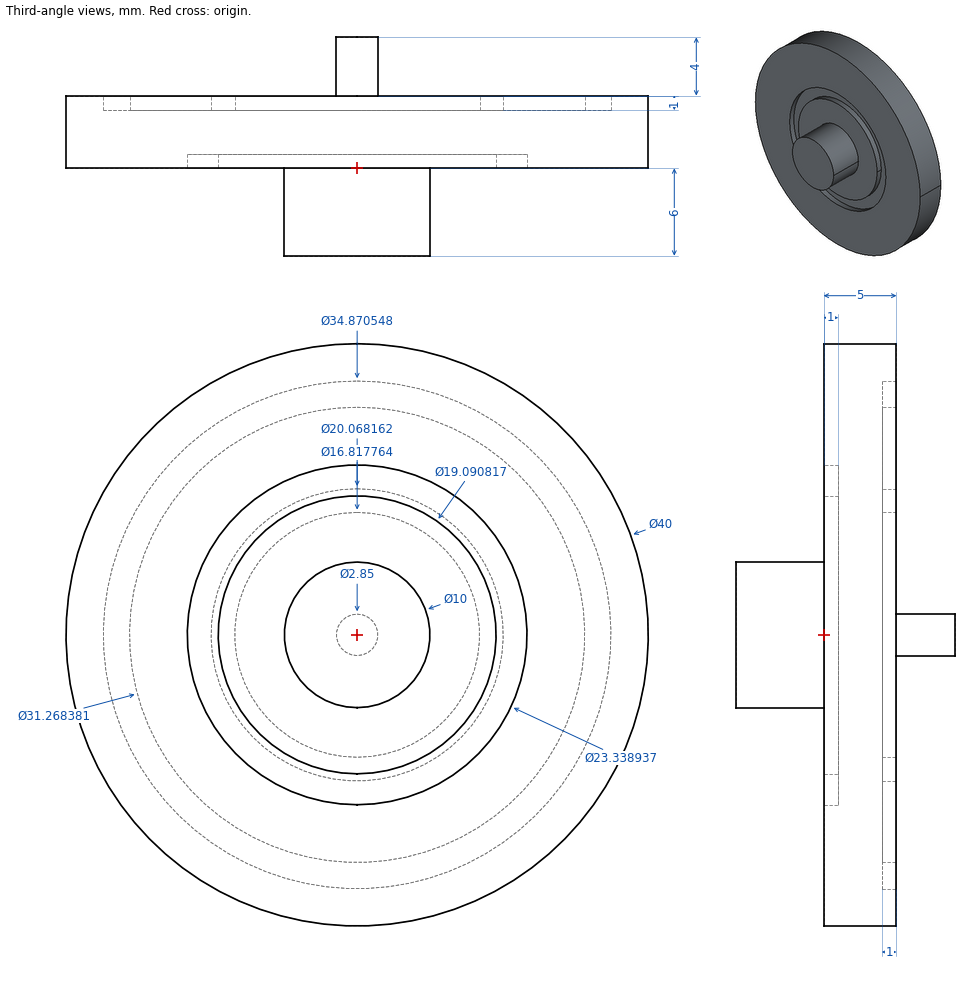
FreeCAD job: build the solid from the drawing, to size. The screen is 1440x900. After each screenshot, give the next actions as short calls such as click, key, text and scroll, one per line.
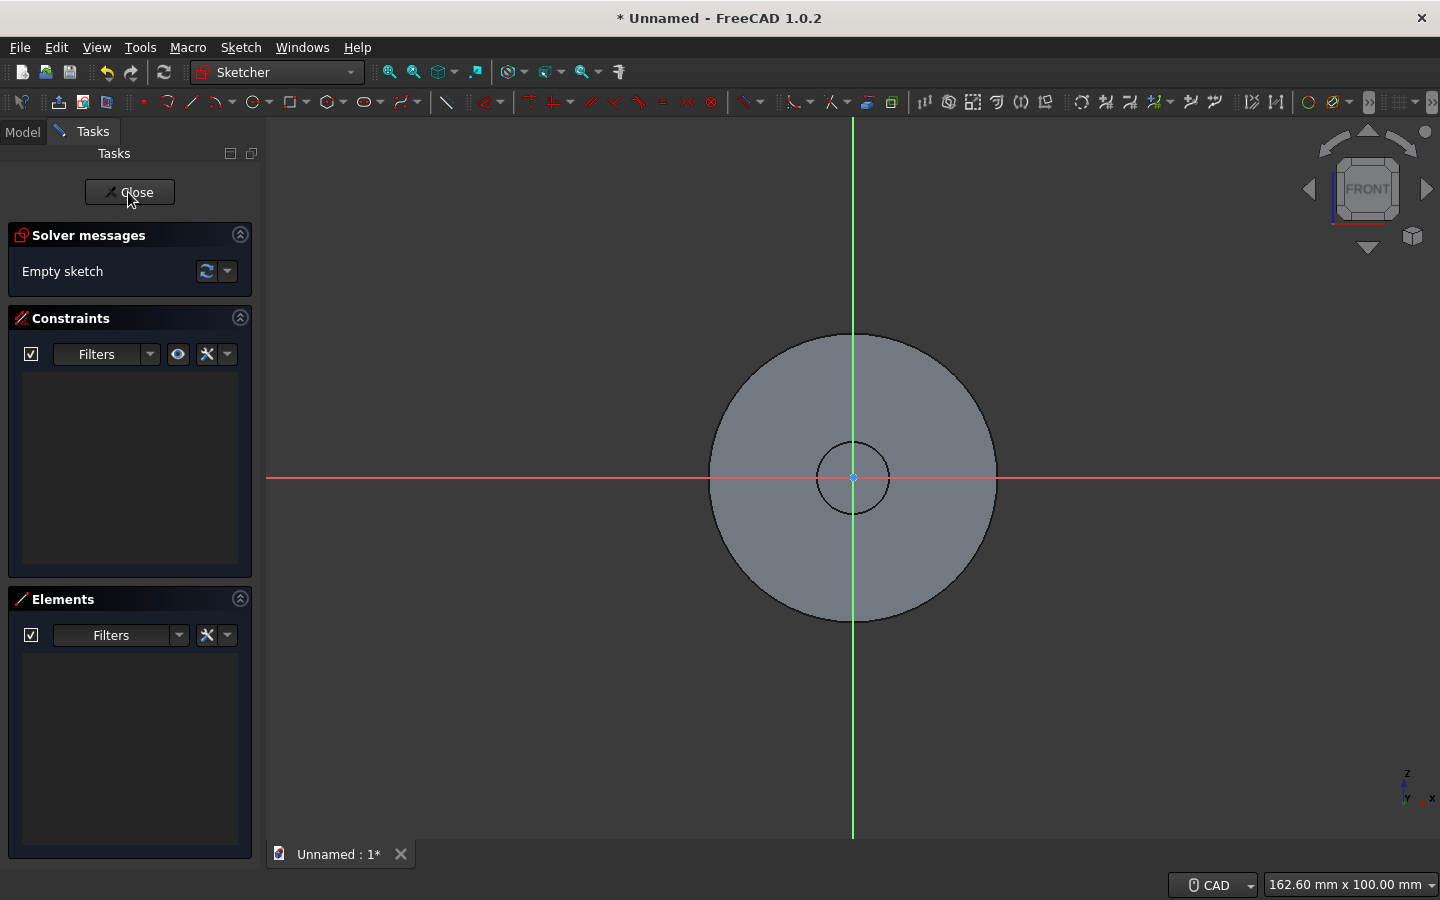
scroll(893, 478, up, 5)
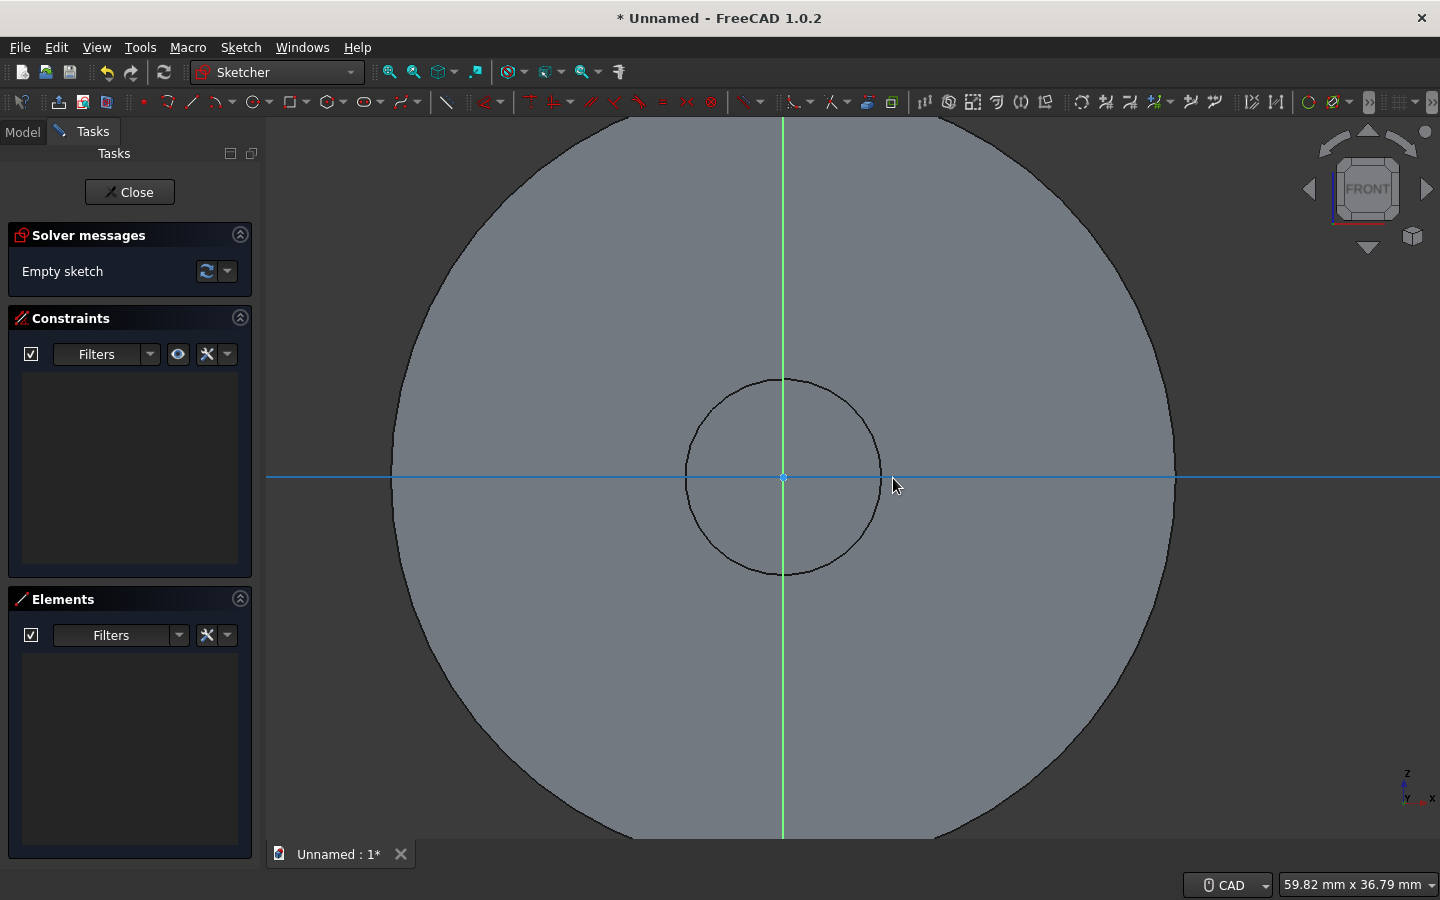
key(g)
key(c)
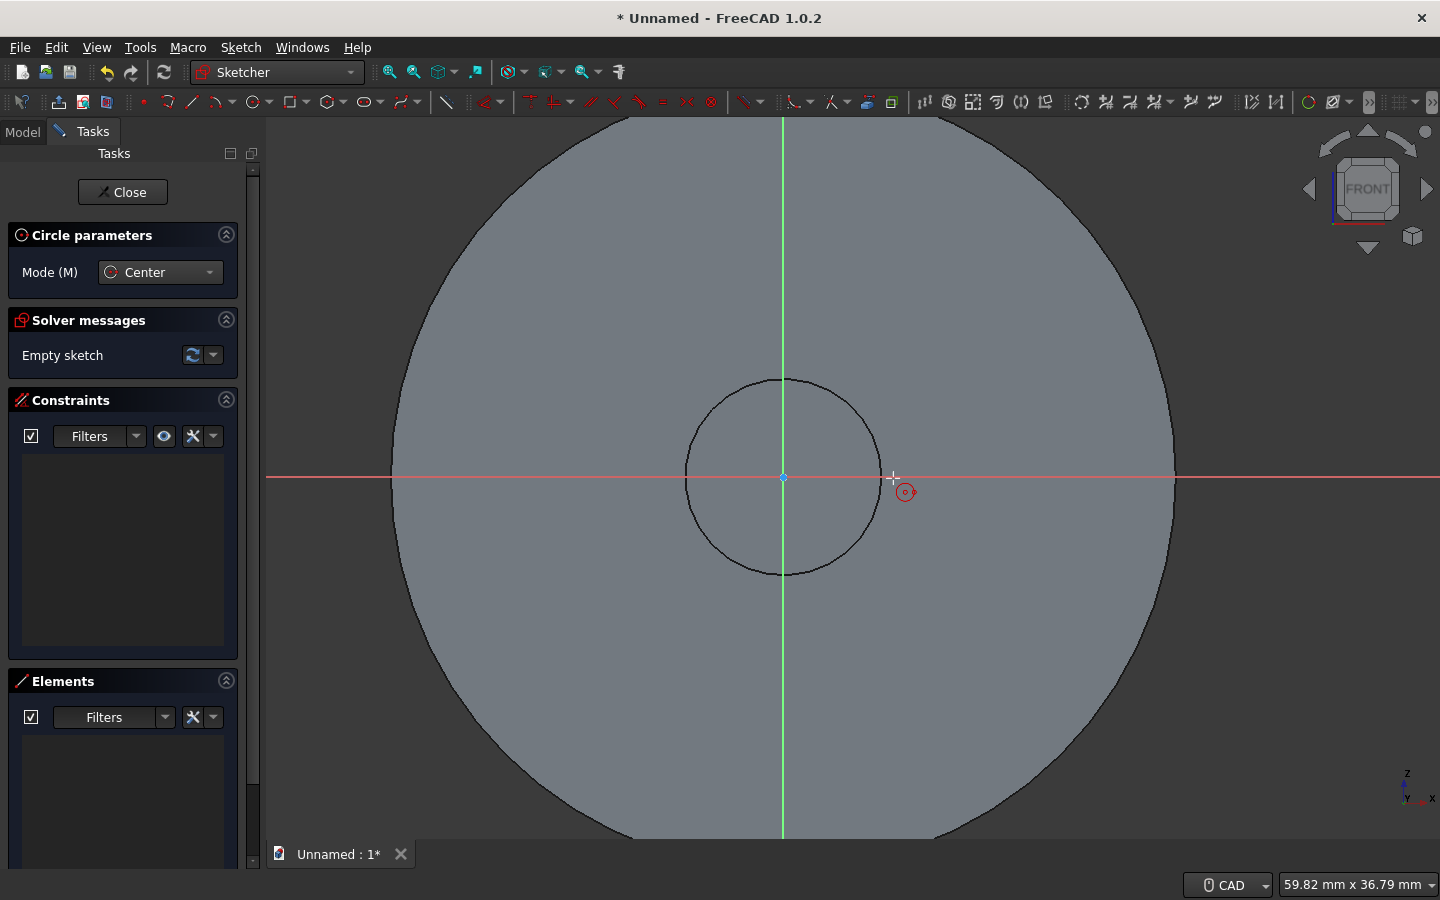
click(783, 477)
click(945, 315)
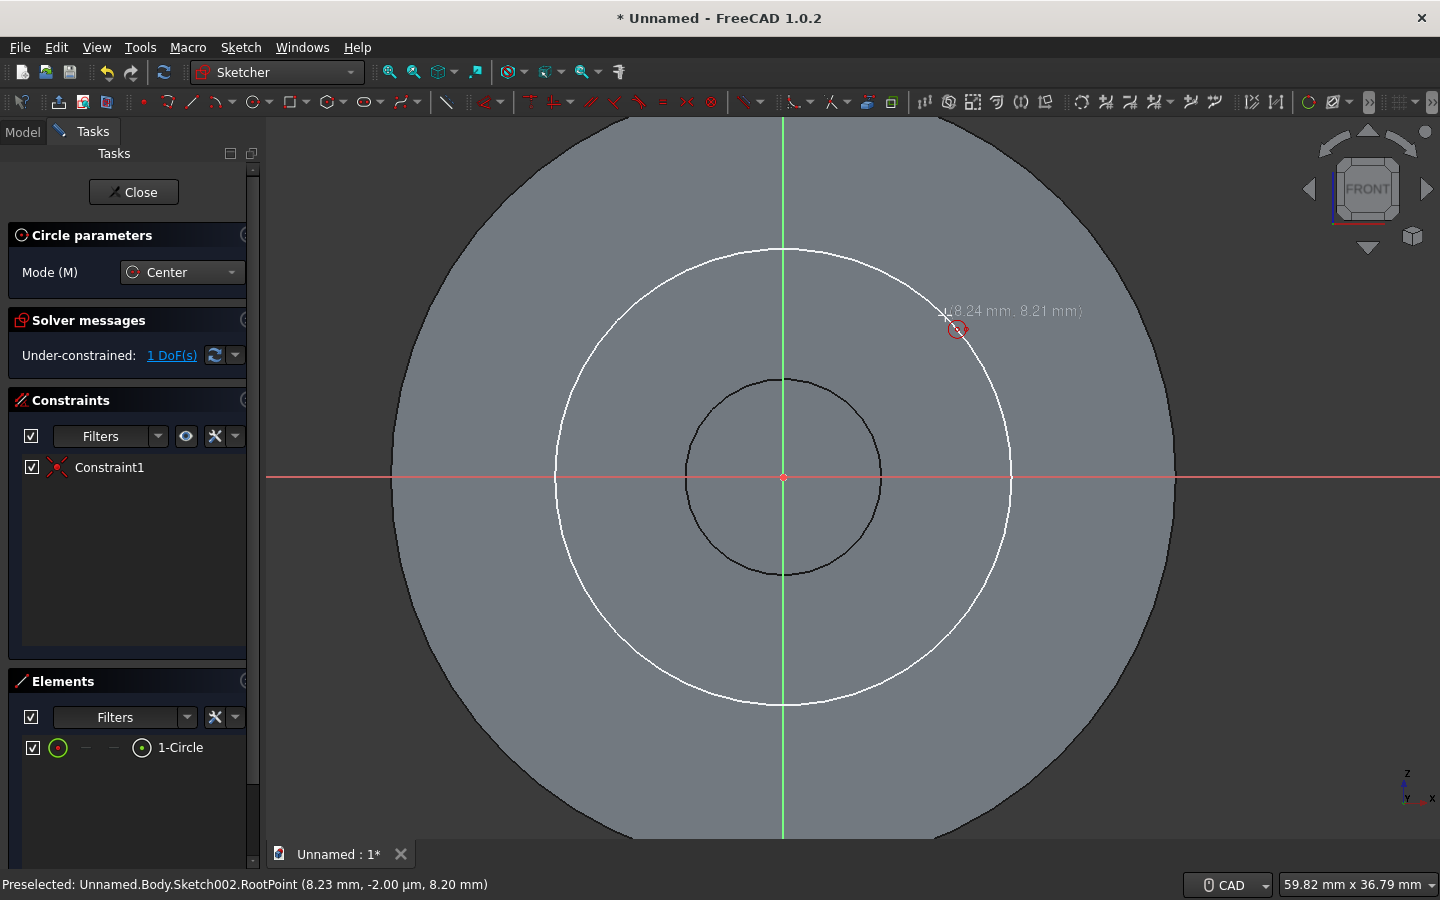
click(783, 477)
click(916, 345)
key(Escape)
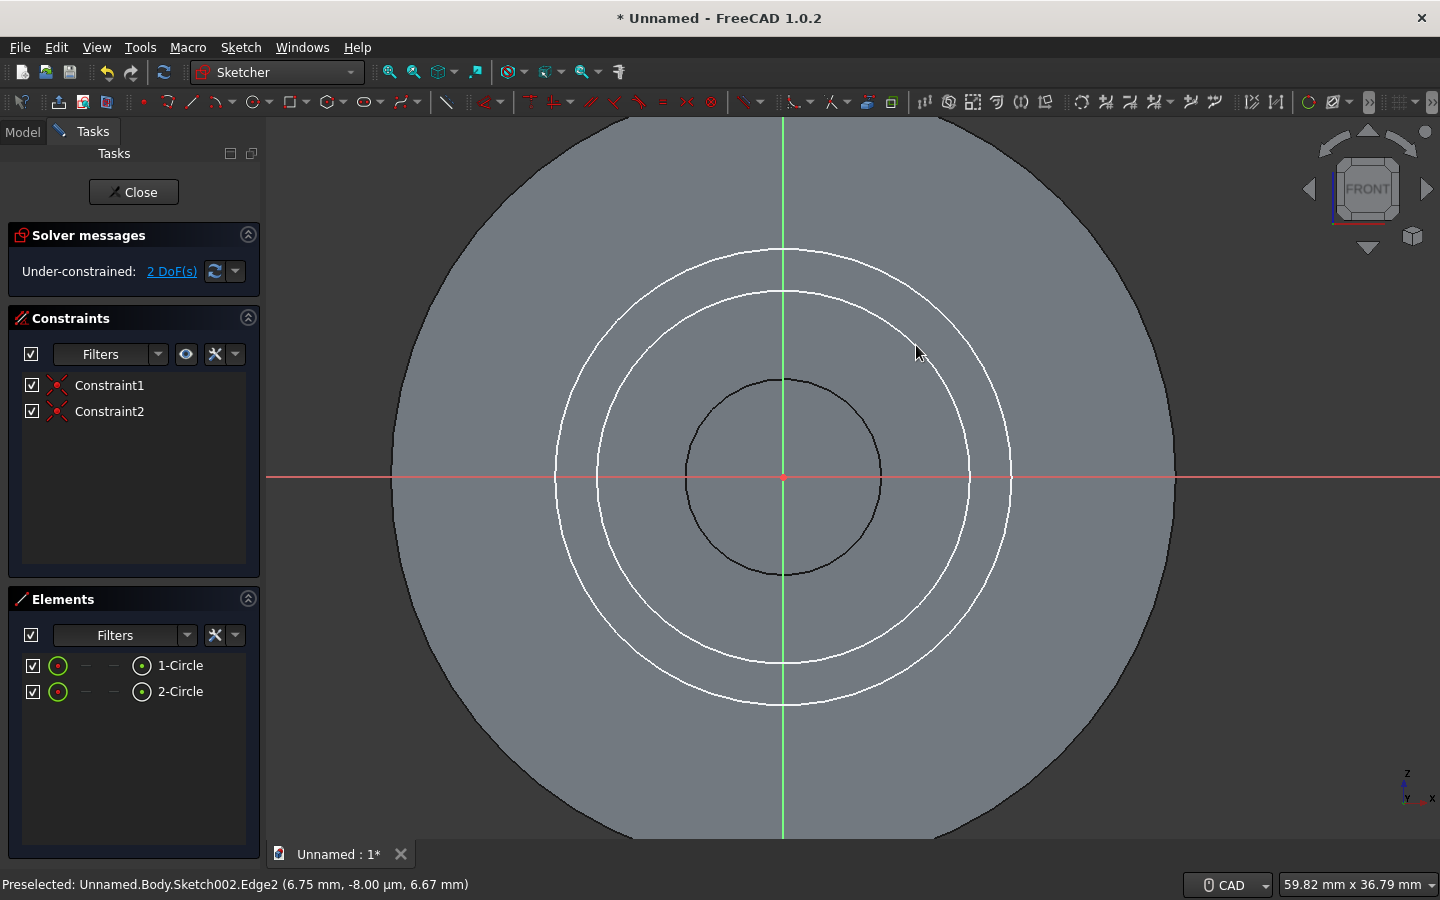
click(484, 102)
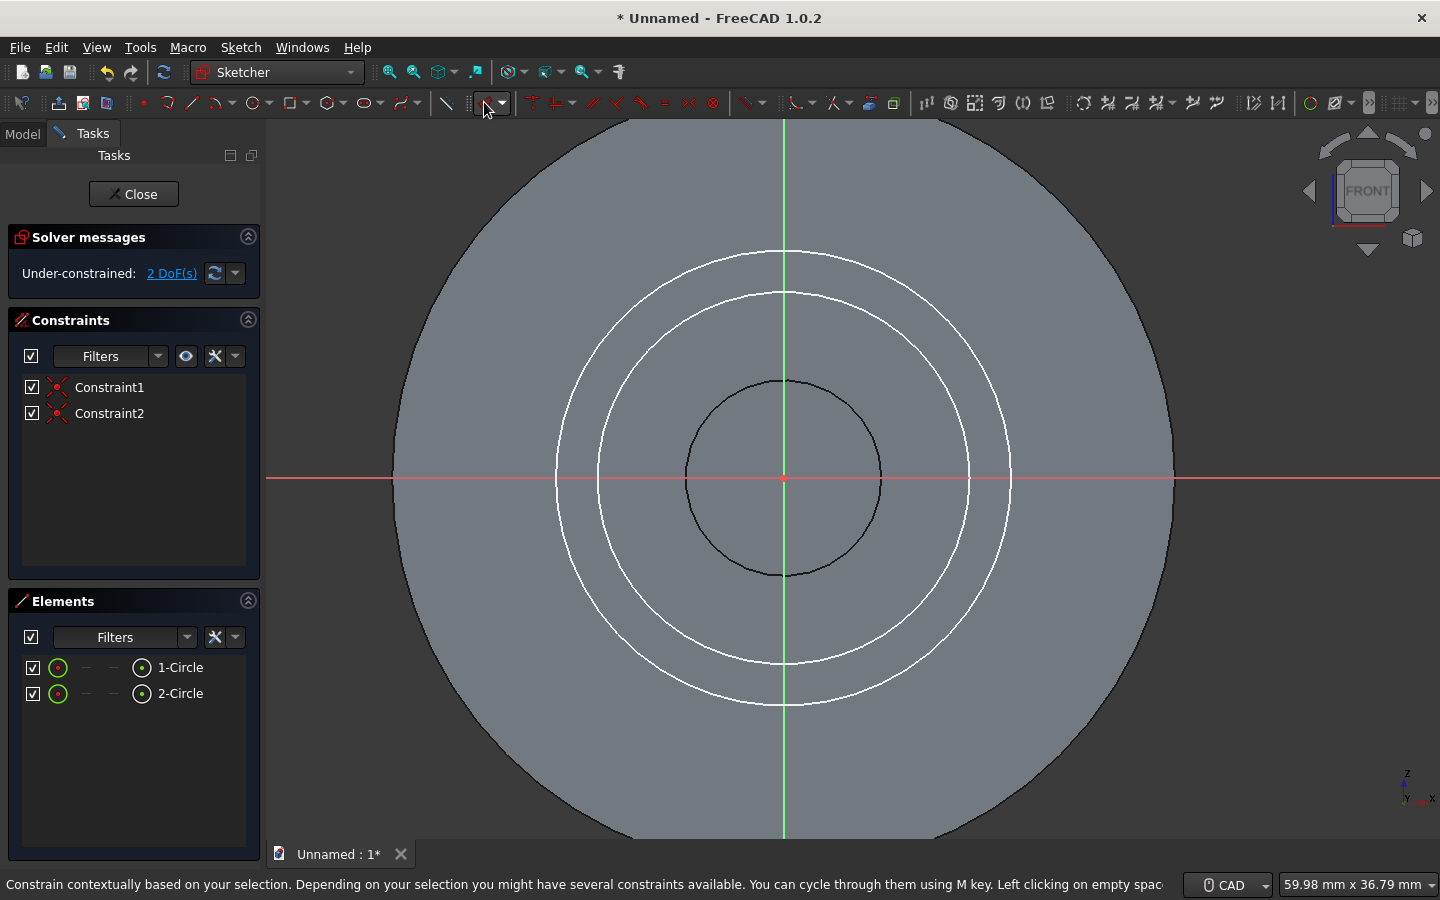
click(944, 317)
click(967, 294)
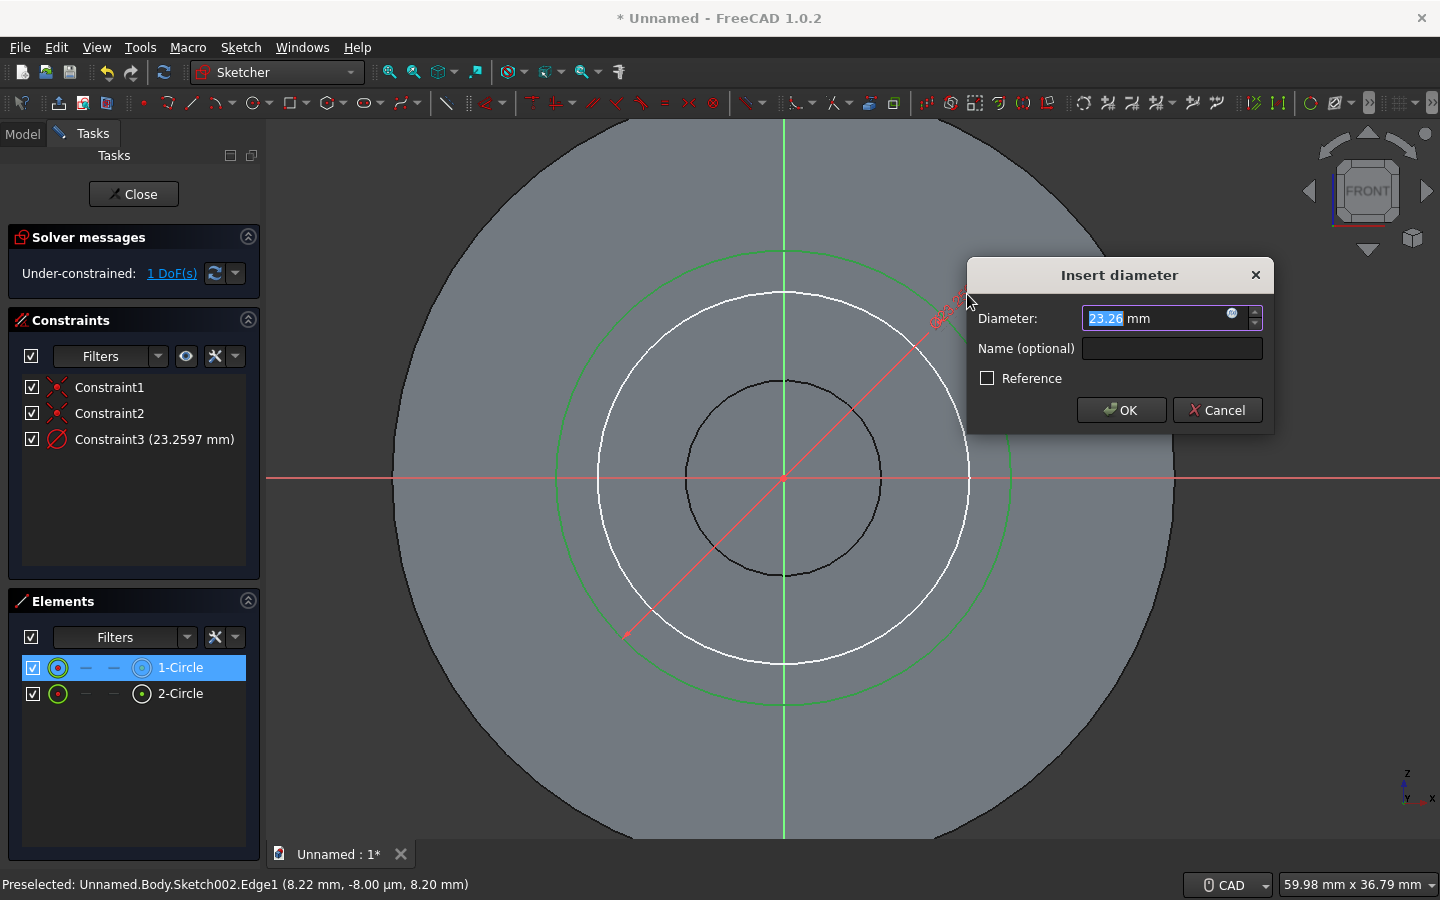
text(23.338937)
key(Return)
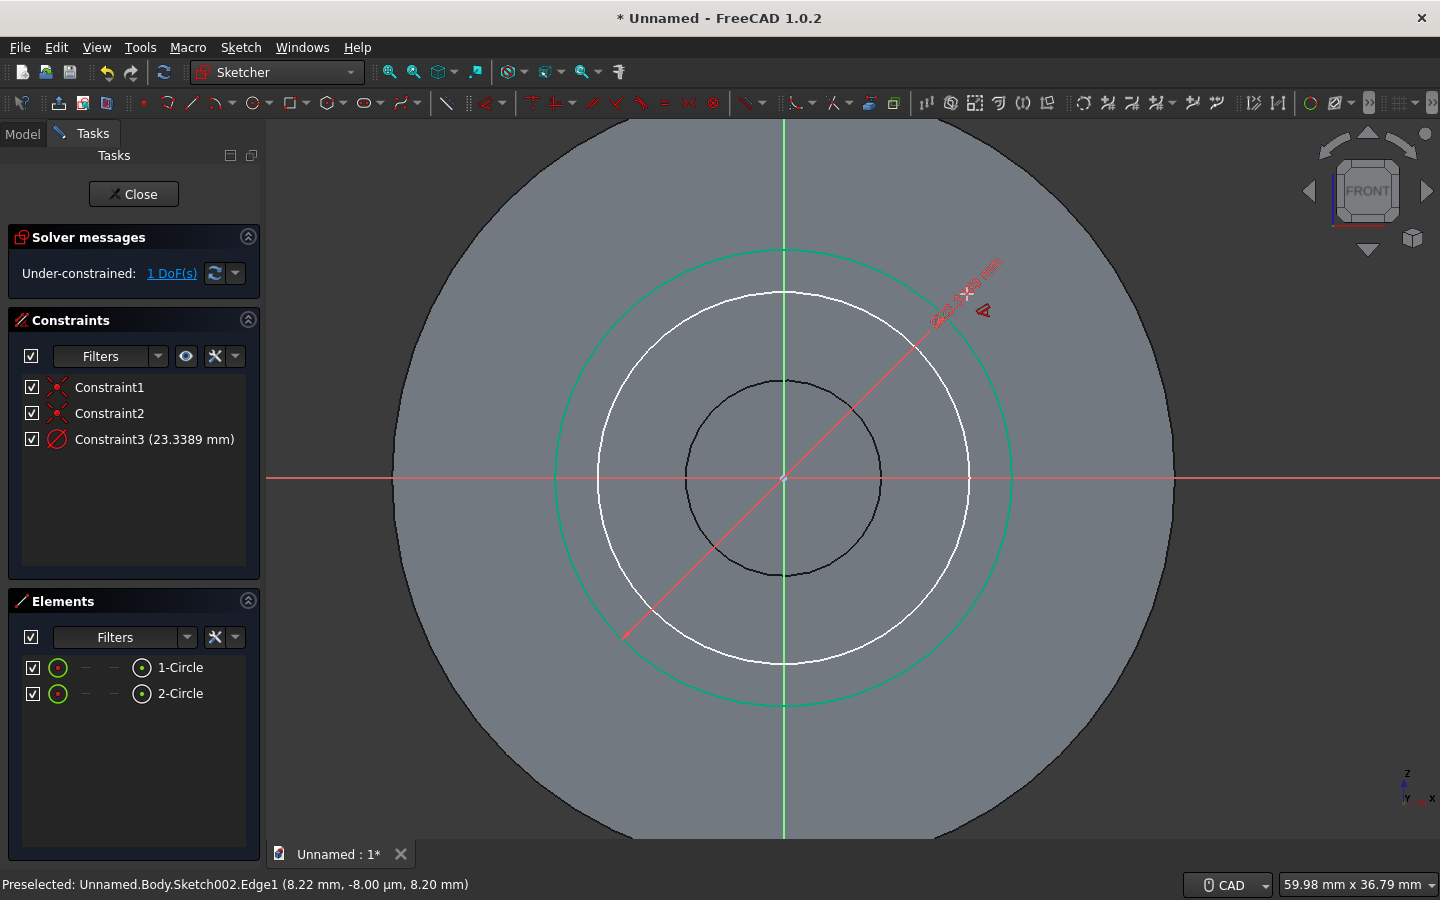
click(915, 346)
click(1015, 410)